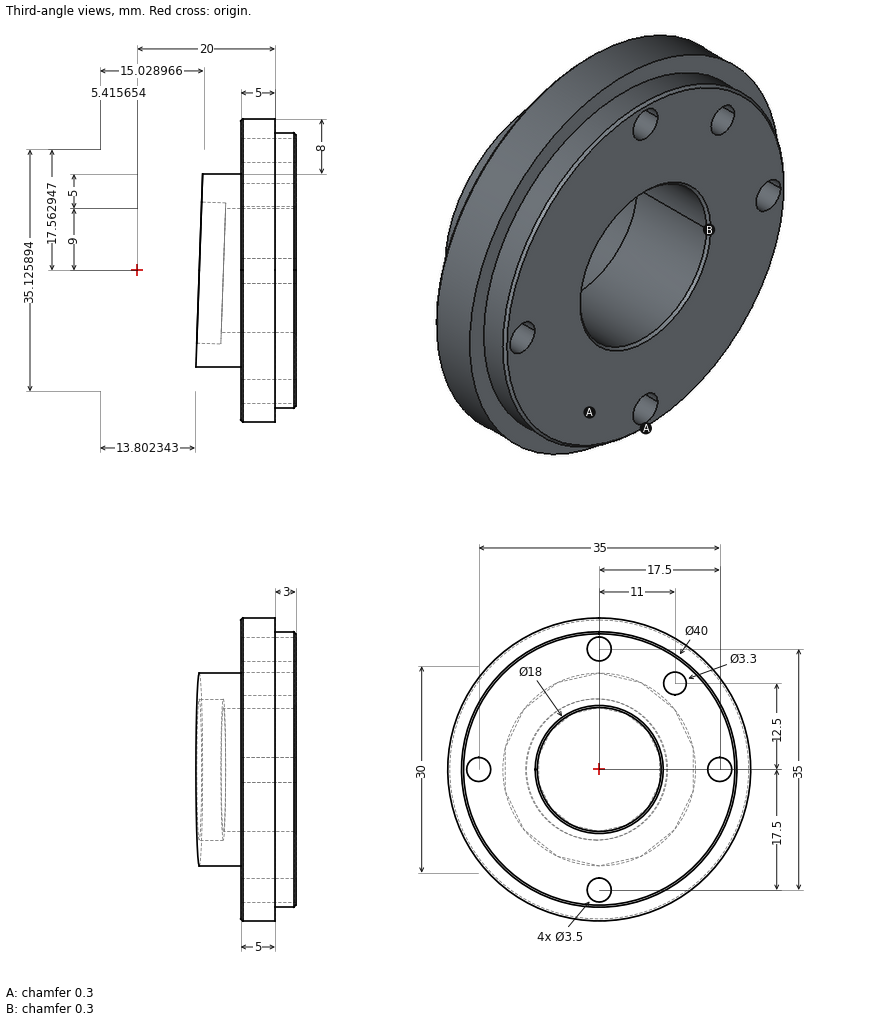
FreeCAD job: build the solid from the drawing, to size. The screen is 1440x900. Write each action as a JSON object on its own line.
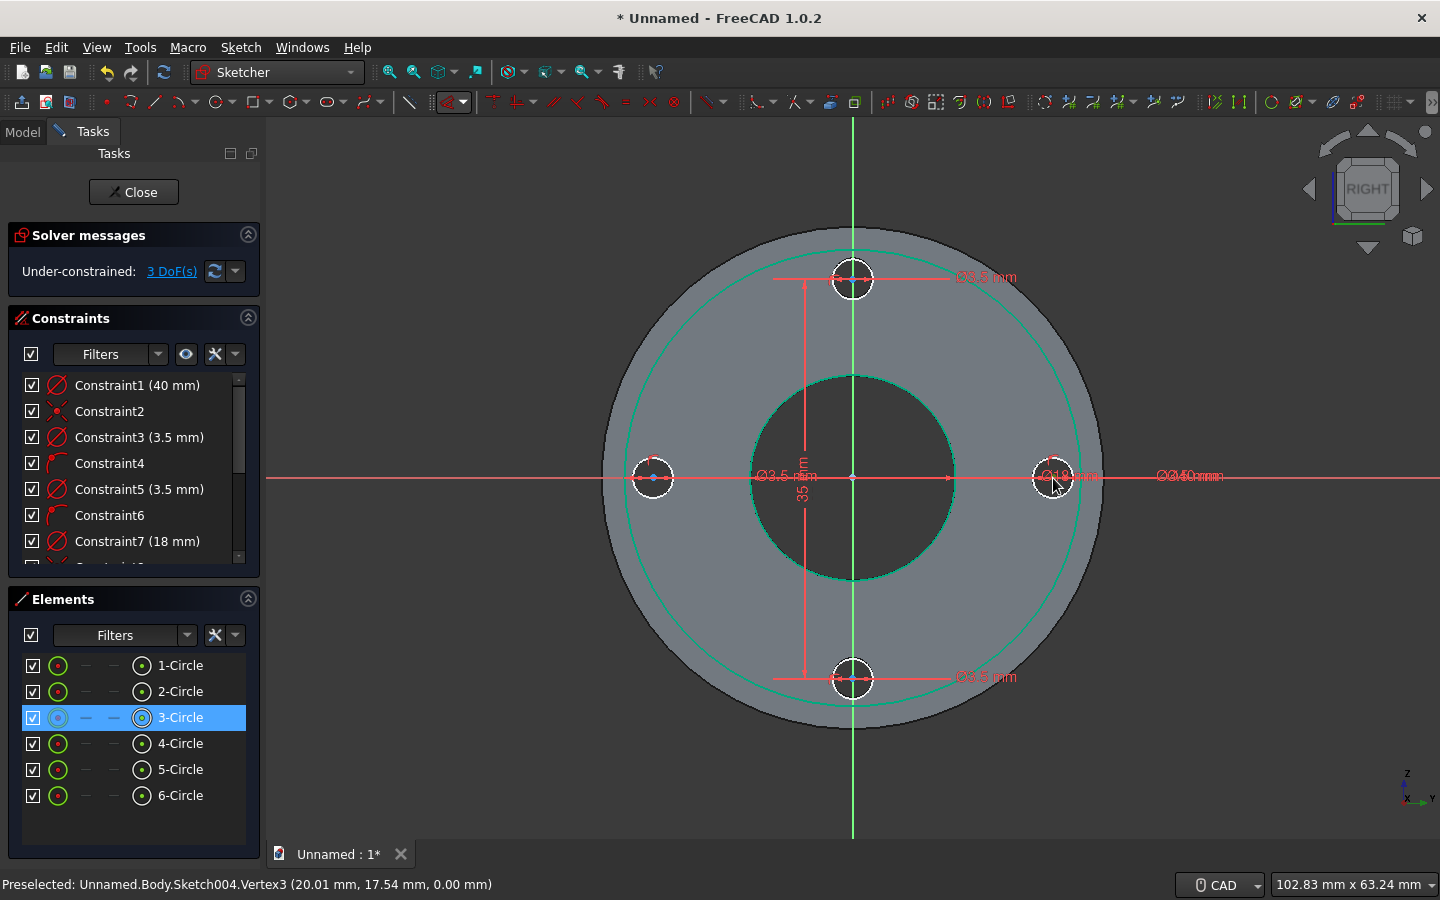
{"action": "left_click", "coordinate": [653, 478]}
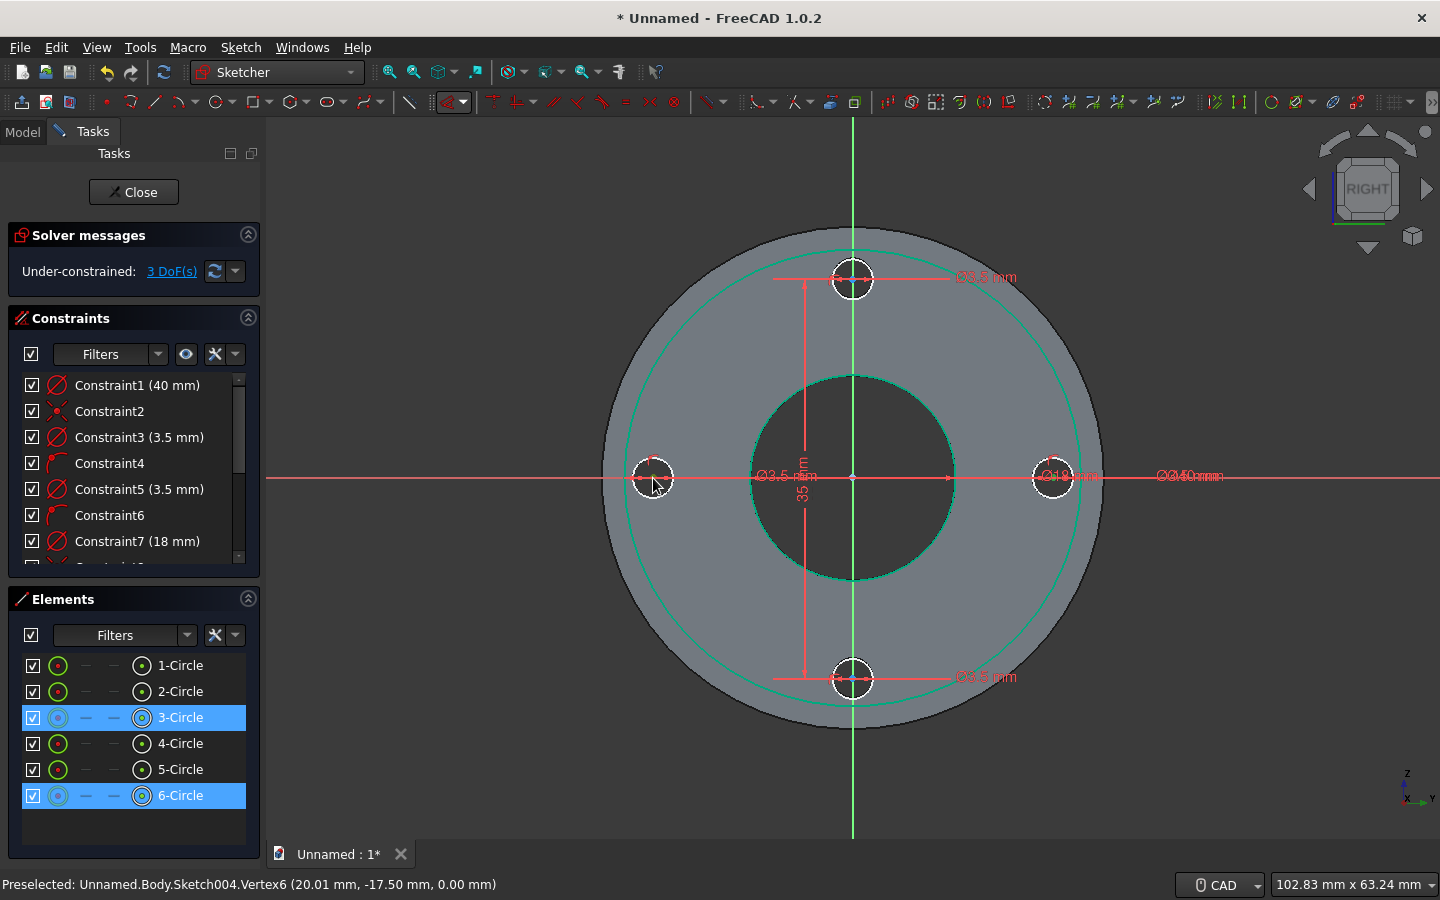
{"action": "left_click", "coordinate": [466, 102]}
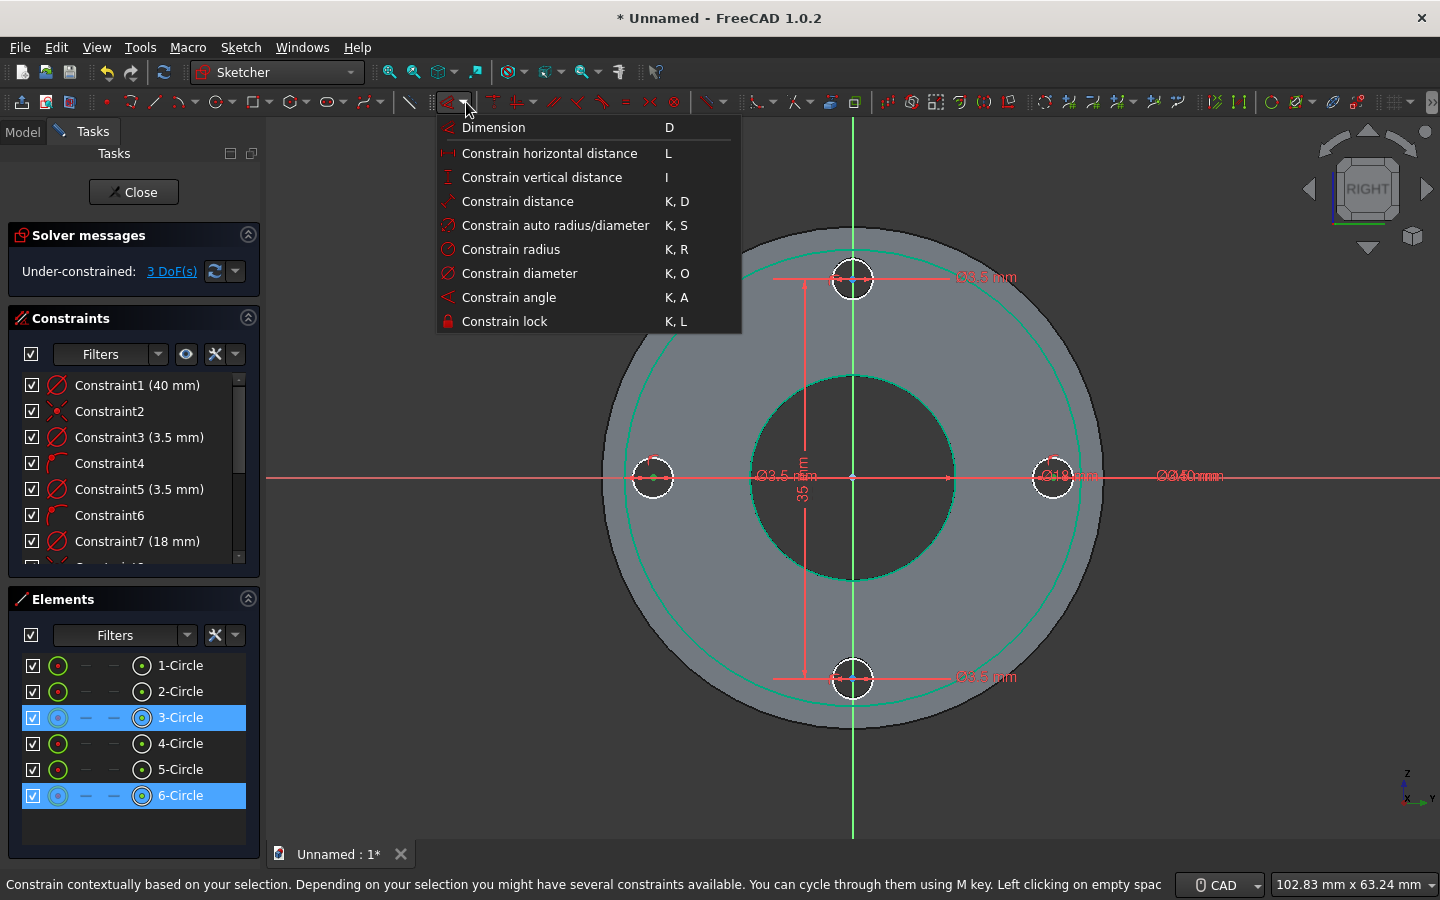
{"action": "left_click", "coordinate": [589, 153]}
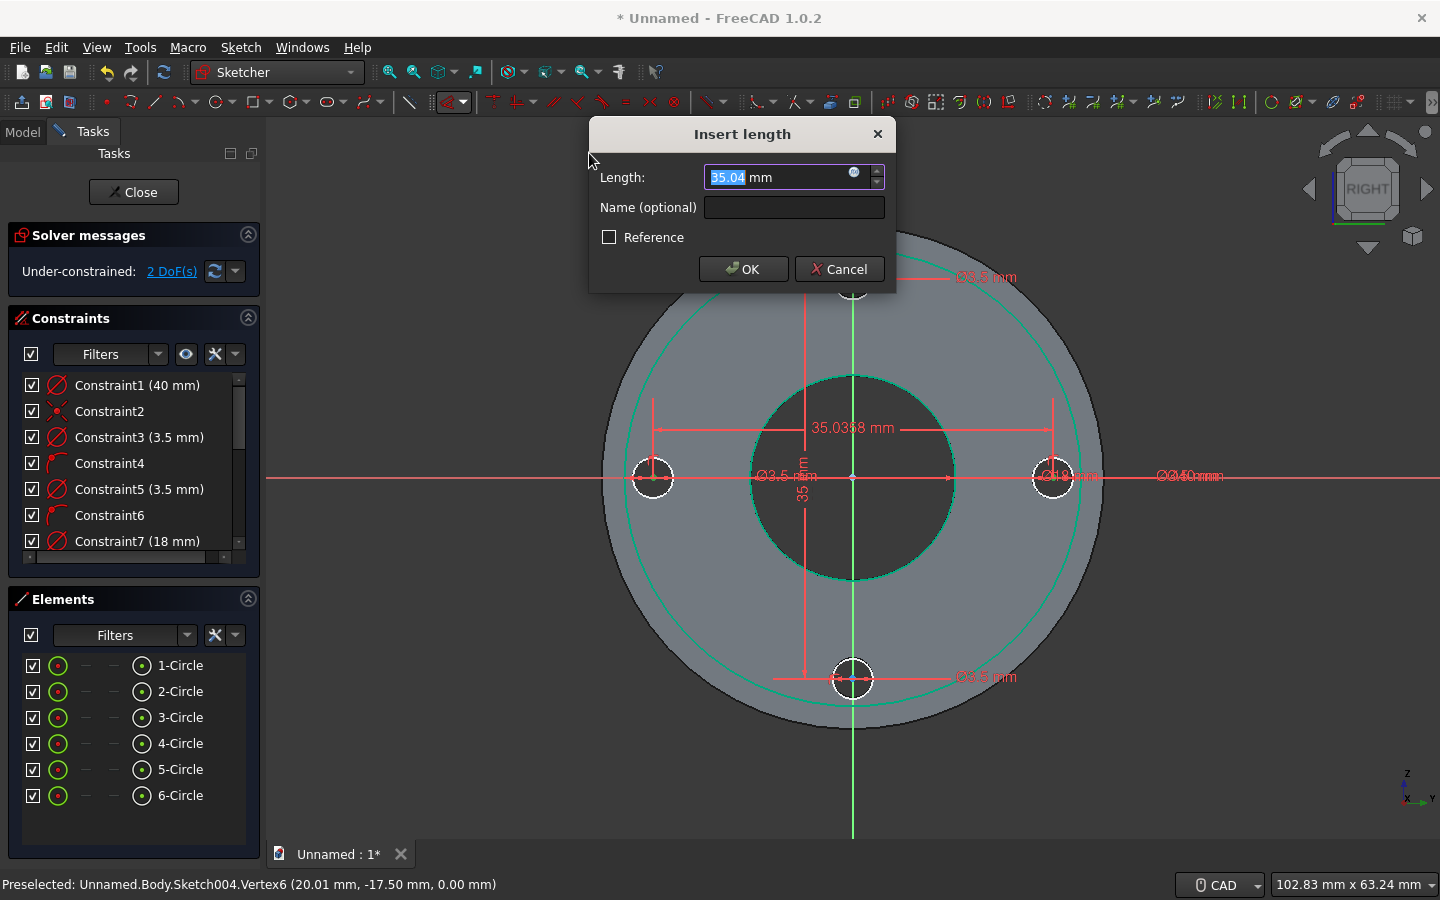
{"action": "type", "text": "35"}
{"action": "key", "text": "Return"}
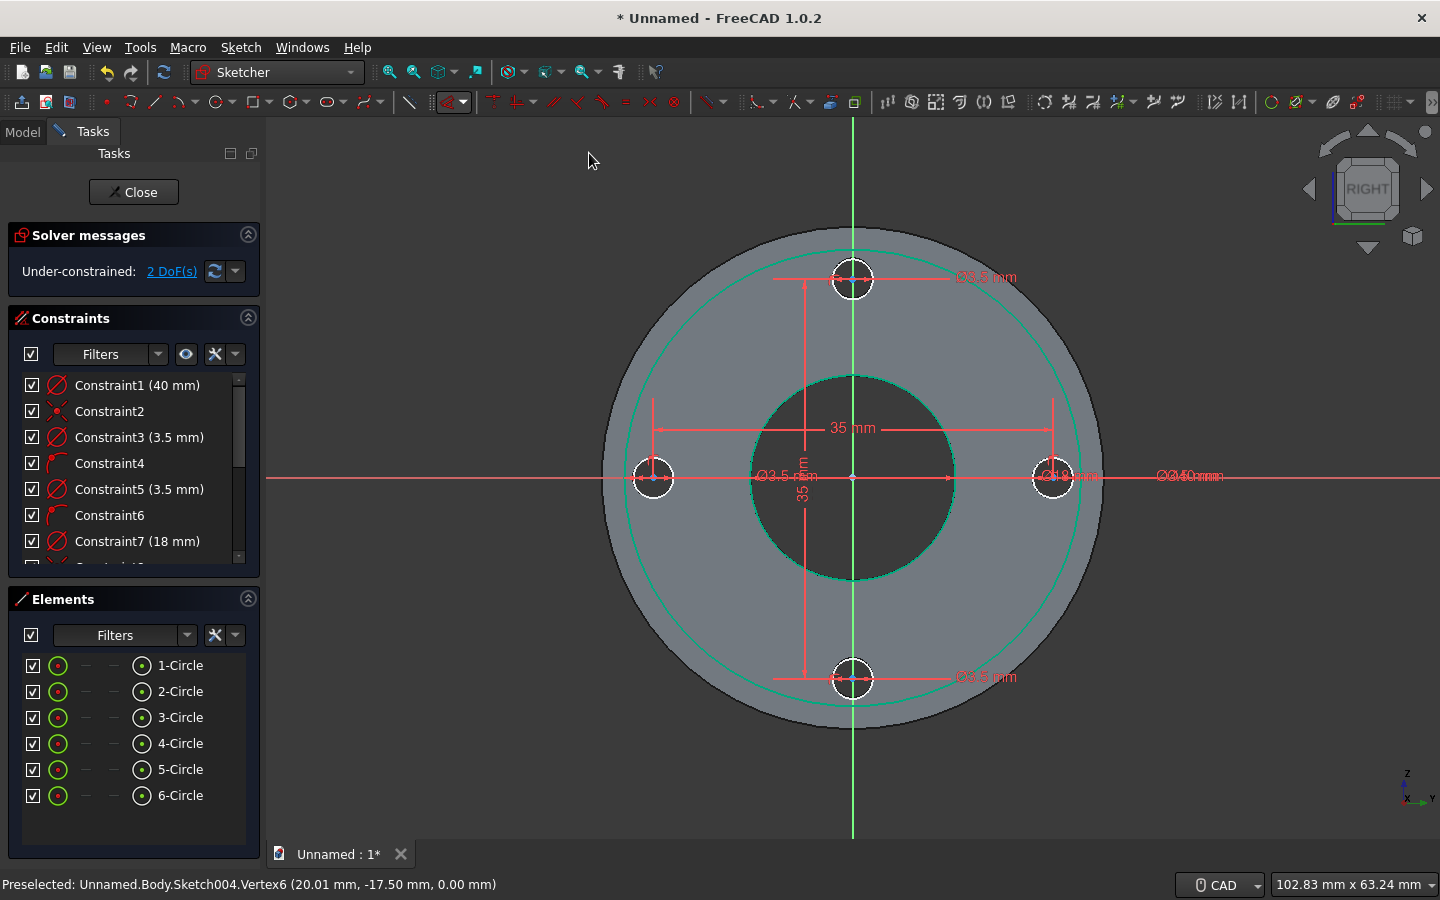
{"action": "left_click", "coordinate": [853, 679]}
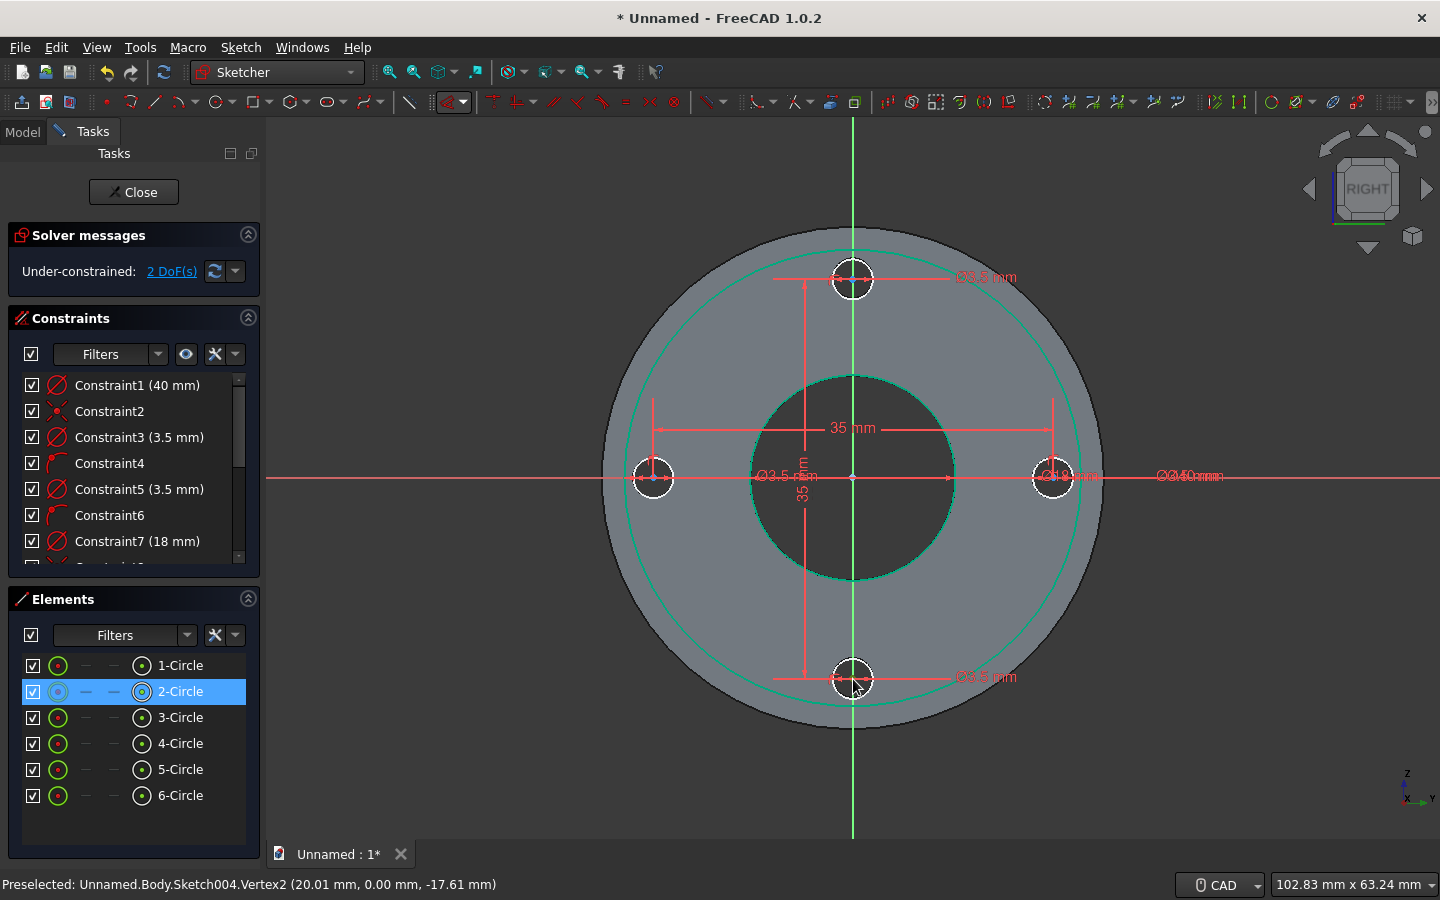
{"action": "left_click", "coordinate": [466, 102]}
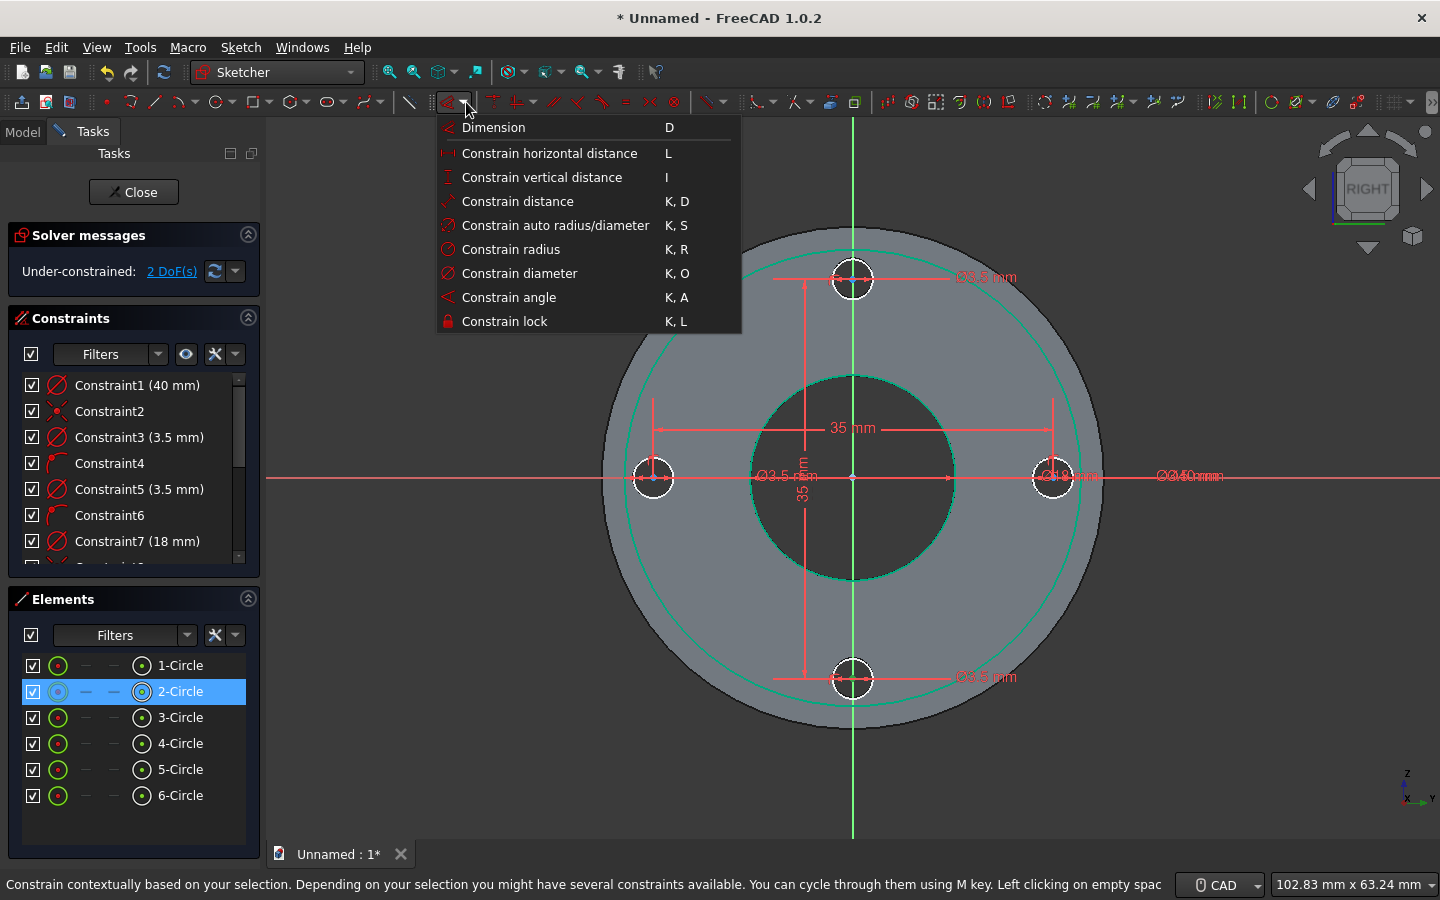
{"action": "left_click", "coordinate": [589, 177]}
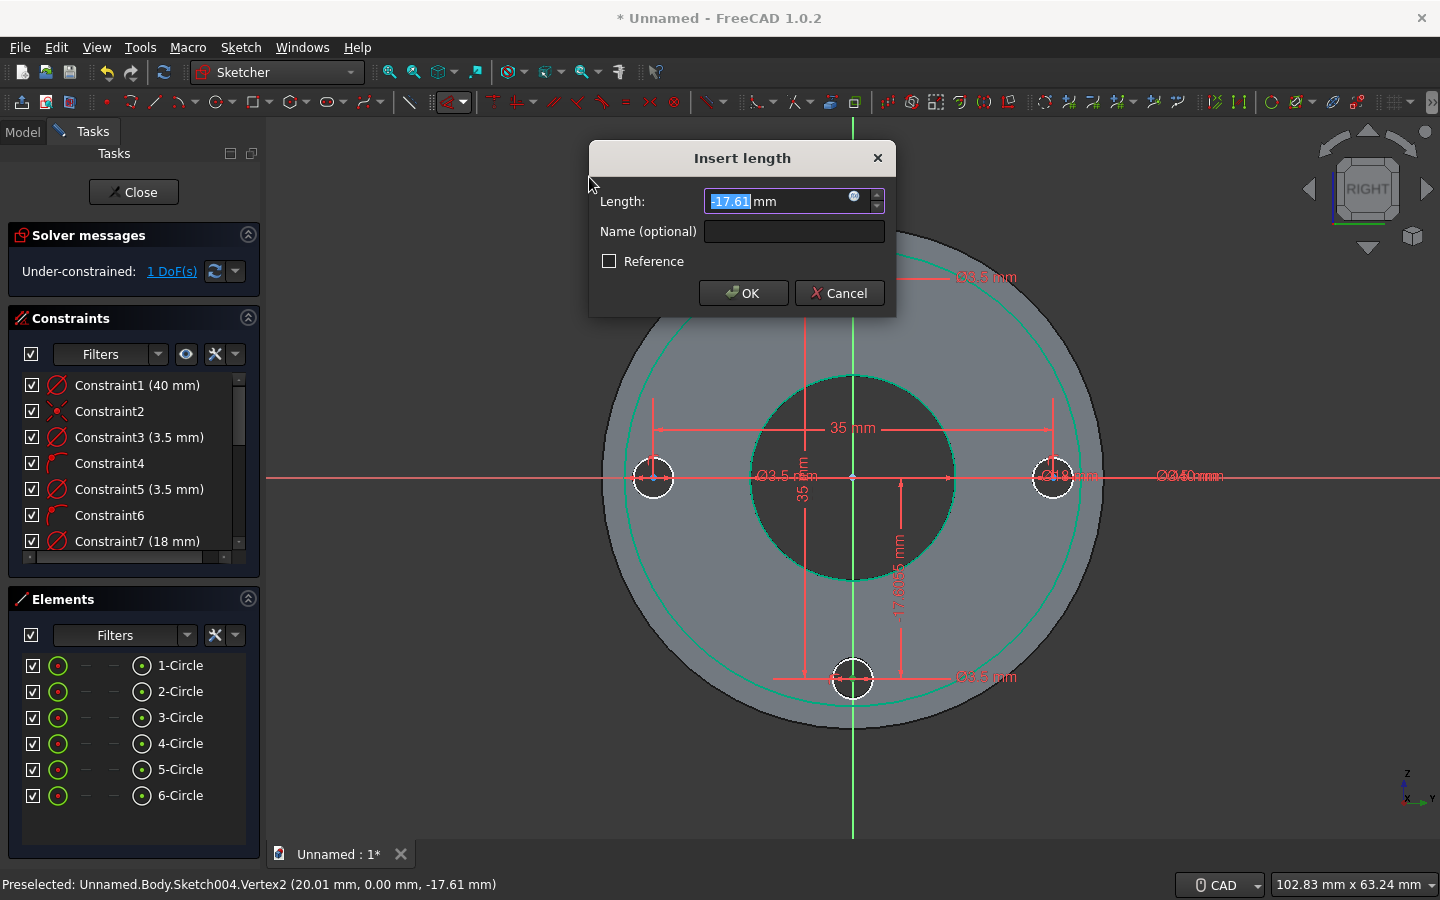
{"action": "type", "text": "-17.5"}
{"action": "key", "text": "Return"}